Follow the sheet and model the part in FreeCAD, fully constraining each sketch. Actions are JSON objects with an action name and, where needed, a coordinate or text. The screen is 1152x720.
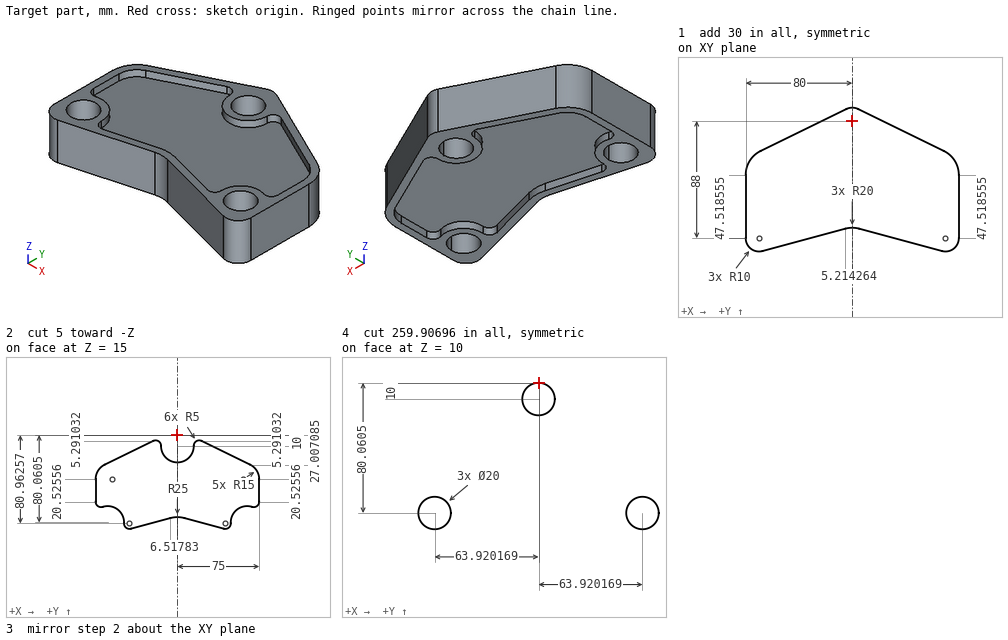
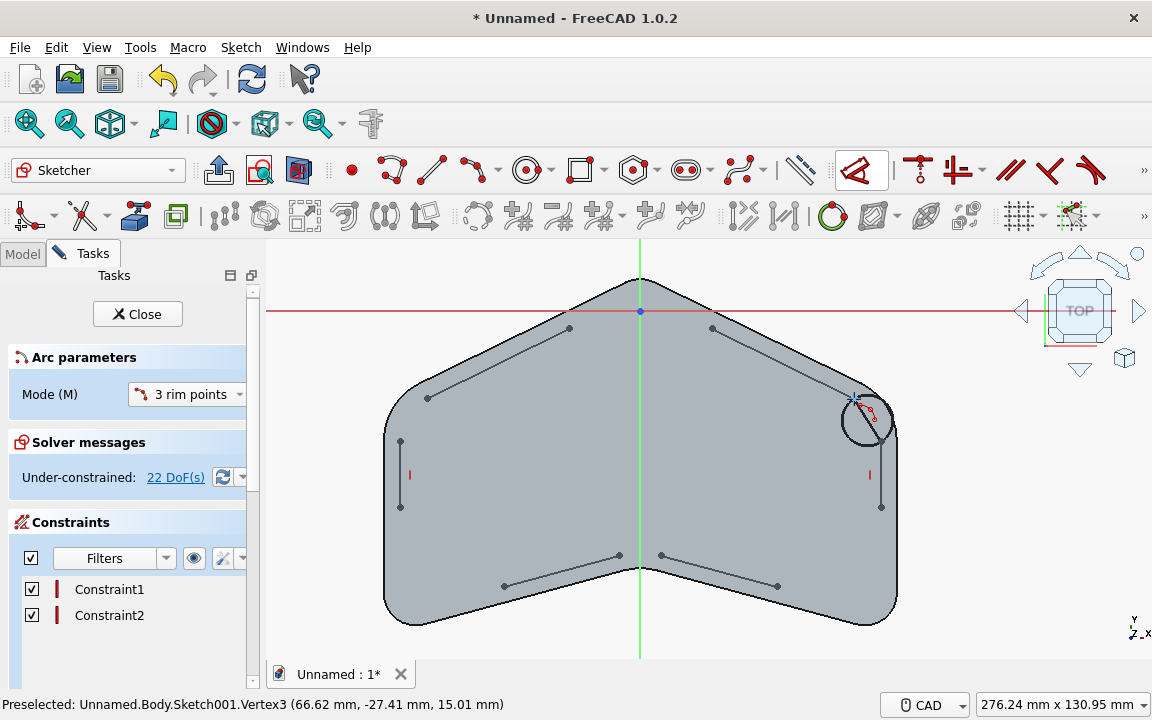
{"action": "scroll", "coordinate": [874, 415], "scroll_direction": "up", "scroll_amount": 4}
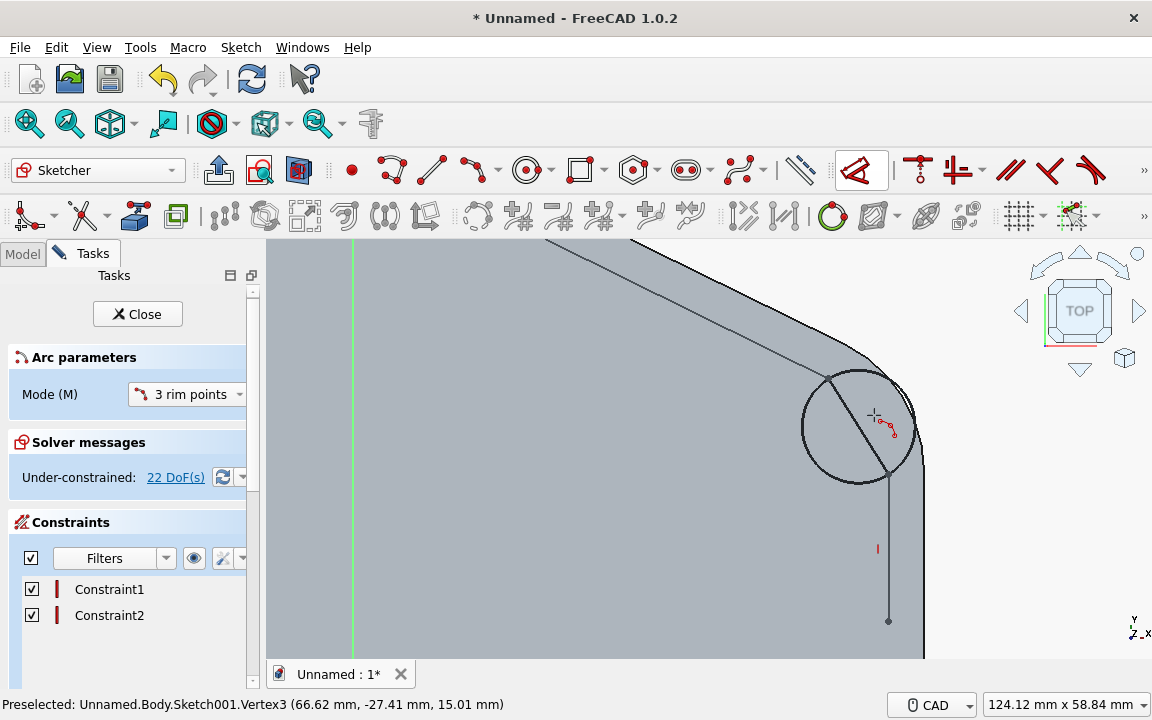
{"action": "left_click", "coordinate": [872, 416]}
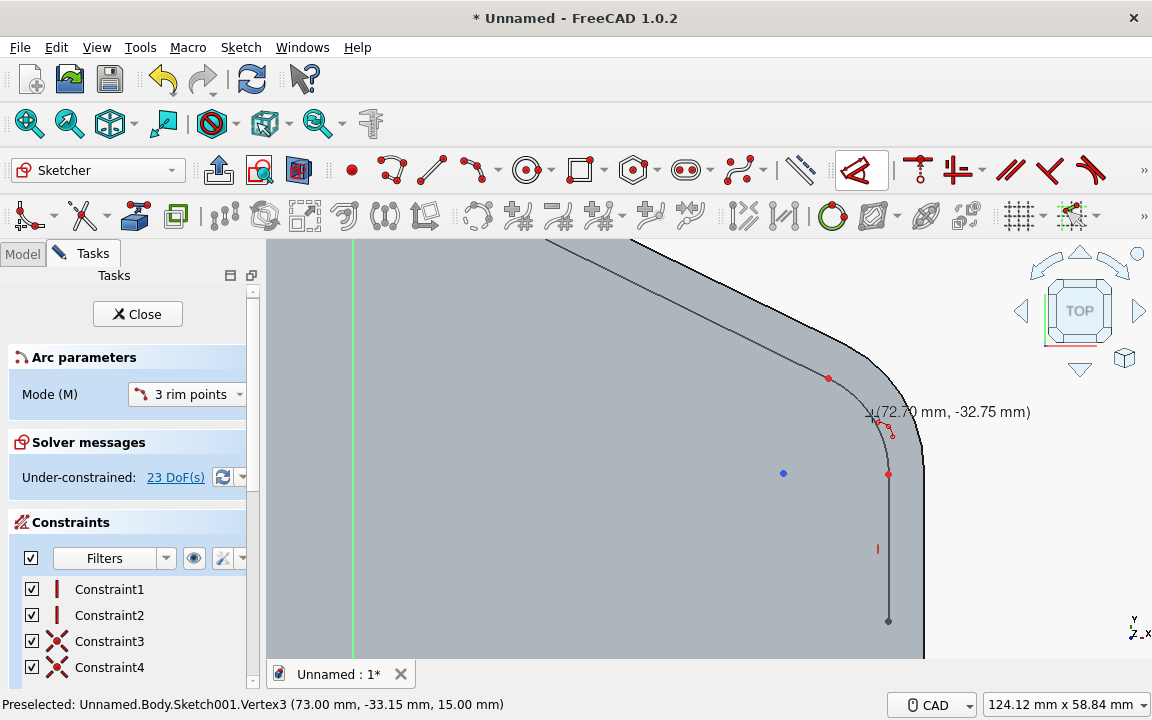
{"action": "scroll", "coordinate": [875, 416], "scroll_direction": "down", "scroll_amount": 4}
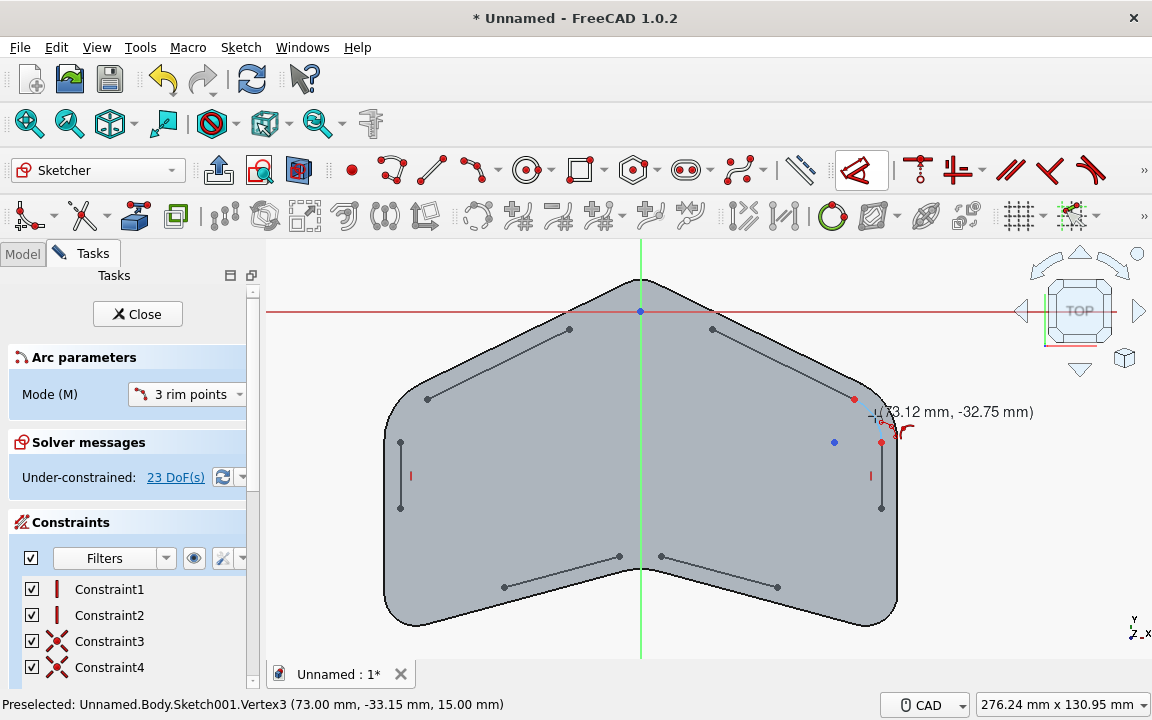
{"action": "left_click", "coordinate": [713, 330]}
{"action": "left_click", "coordinate": [689, 343]}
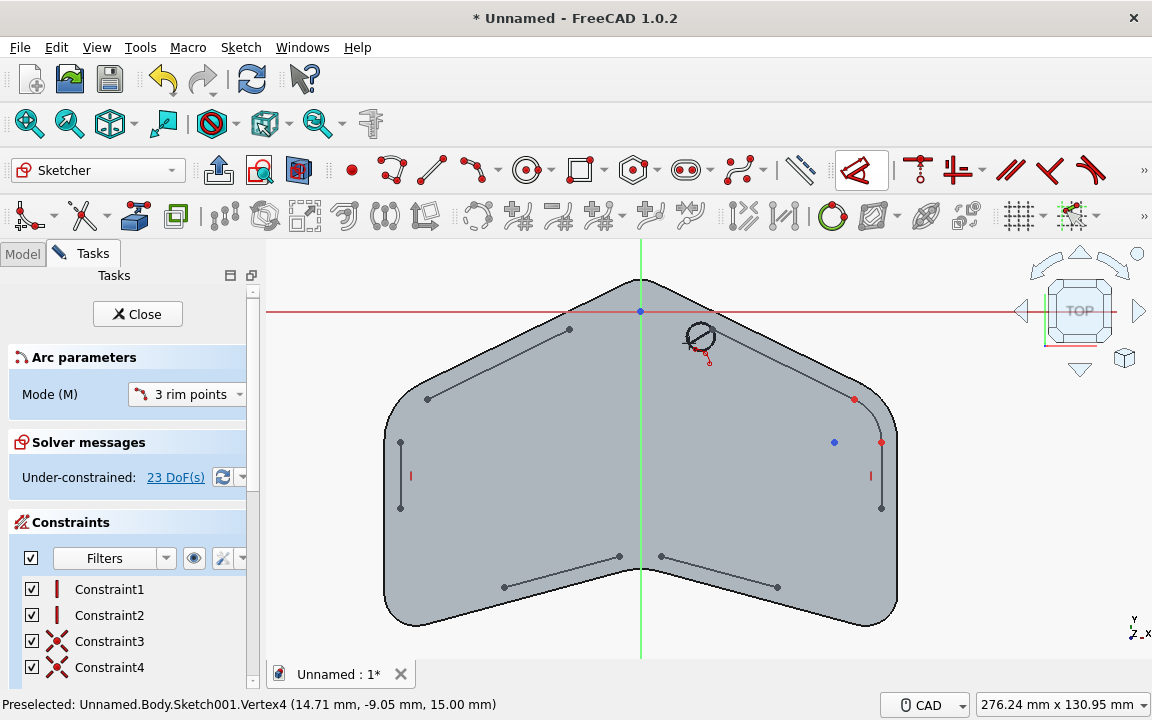
{"action": "scroll", "coordinate": [696, 329], "scroll_direction": "up", "scroll_amount": 4}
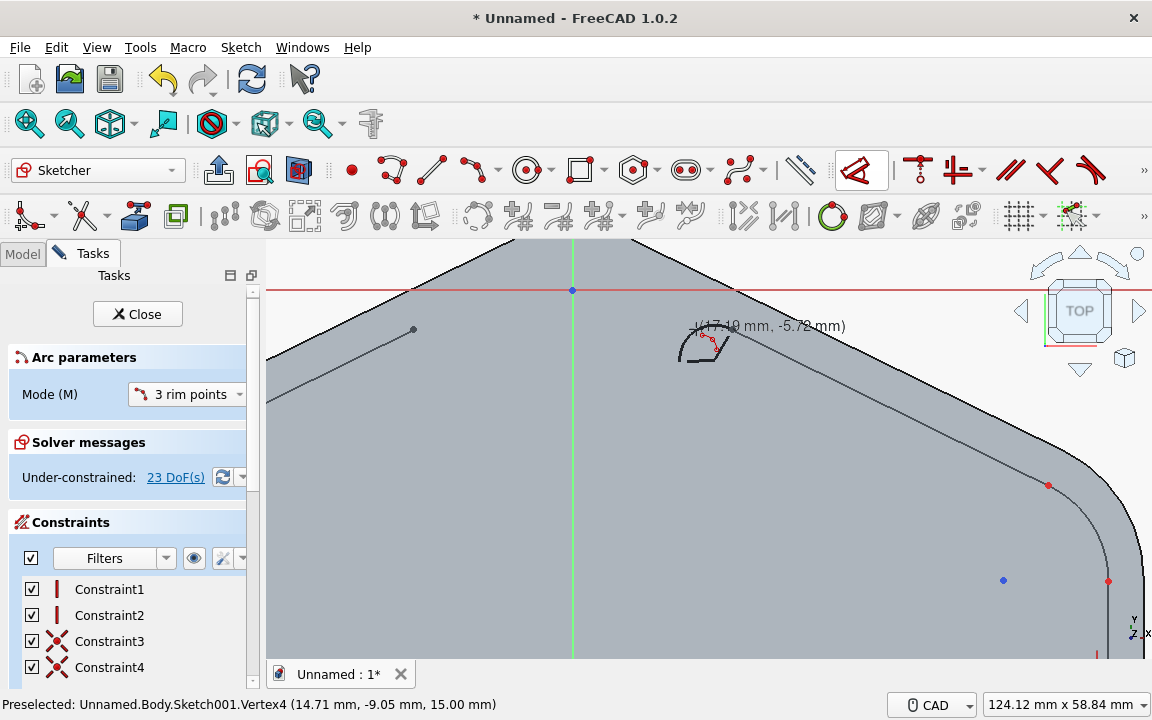
{"action": "left_click", "coordinate": [696, 330]}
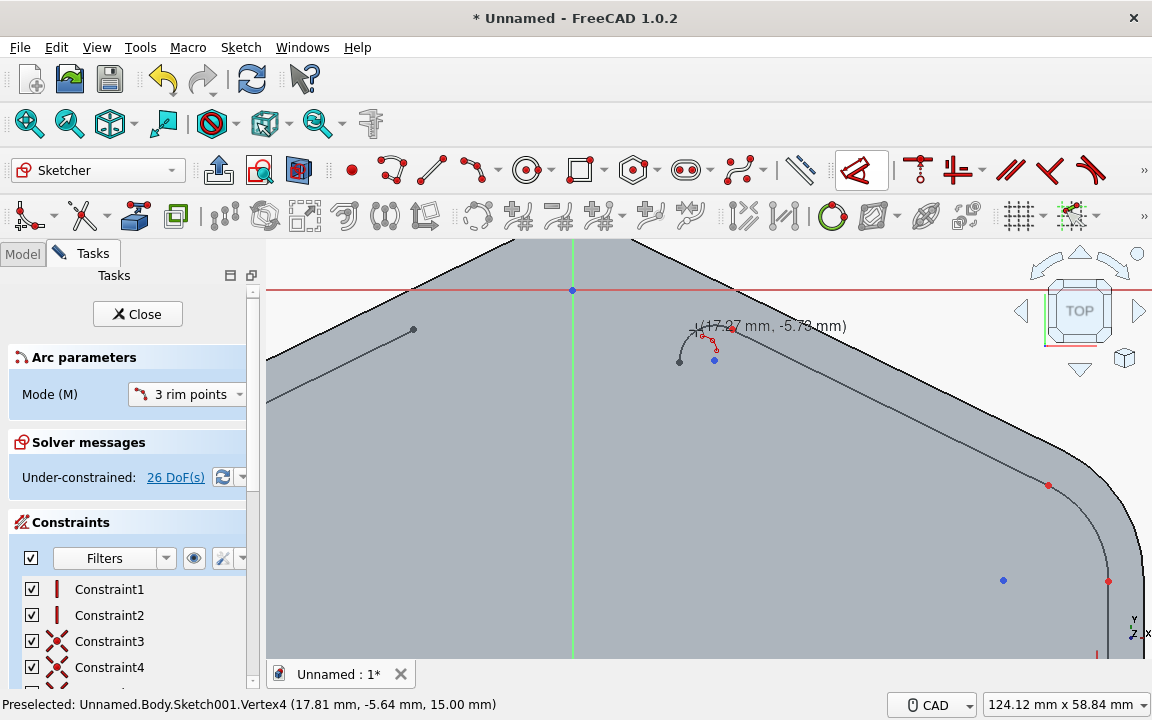
{"action": "left_click", "coordinate": [680, 362]}
{"action": "left_click", "coordinate": [466, 360]}
{"action": "left_click", "coordinate": [539, 463]}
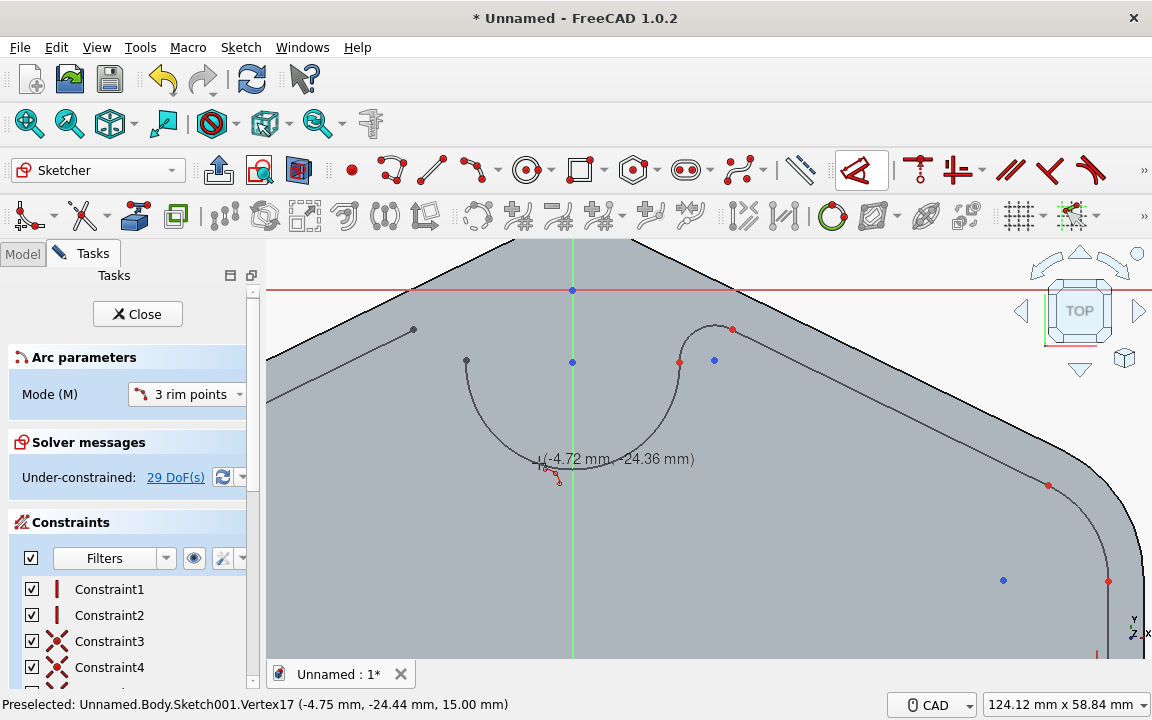
{"action": "left_click", "coordinate": [466, 361]}
{"action": "left_click", "coordinate": [414, 330]}
{"action": "left_click", "coordinate": [449, 330]}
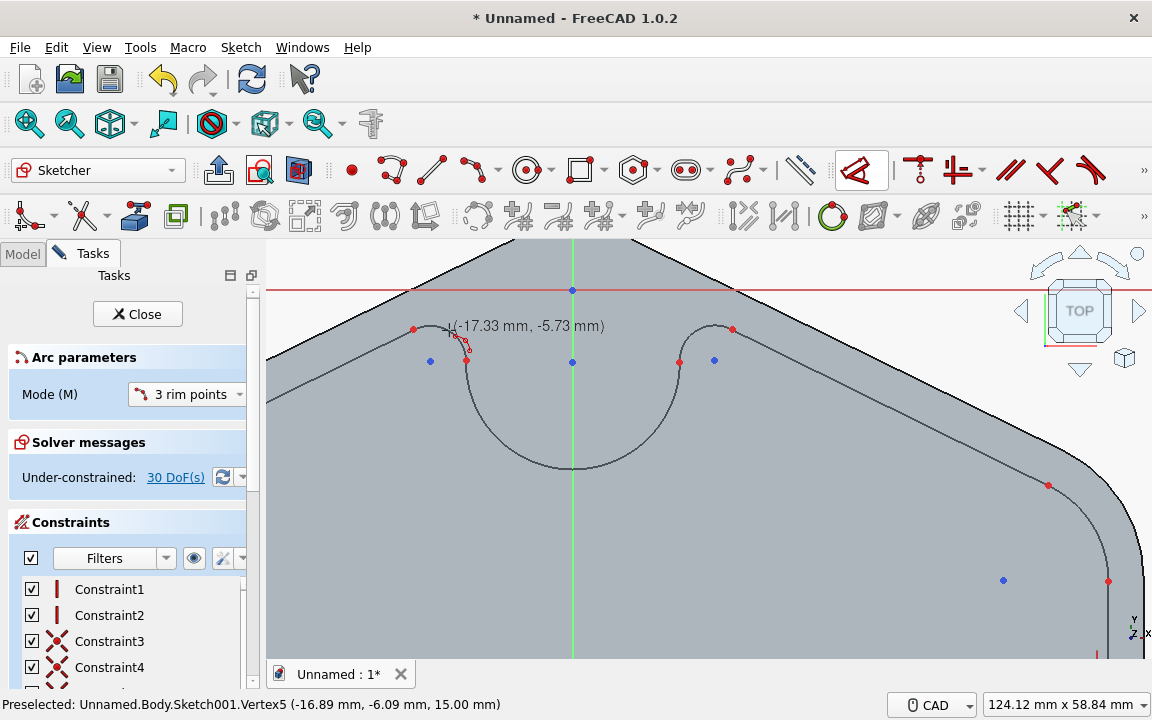
{"action": "scroll", "coordinate": [696, 329], "scroll_direction": "down", "scroll_amount": 4}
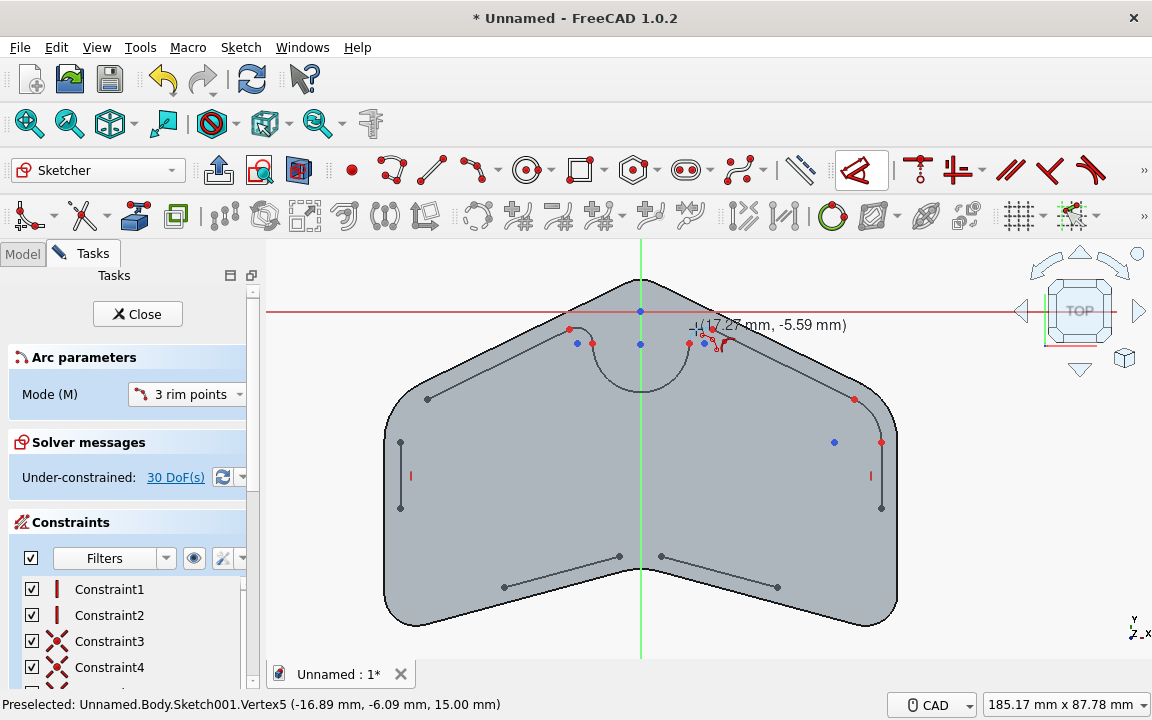
{"action": "left_click", "coordinate": [428, 400]}
{"action": "left_click", "coordinate": [401, 443]}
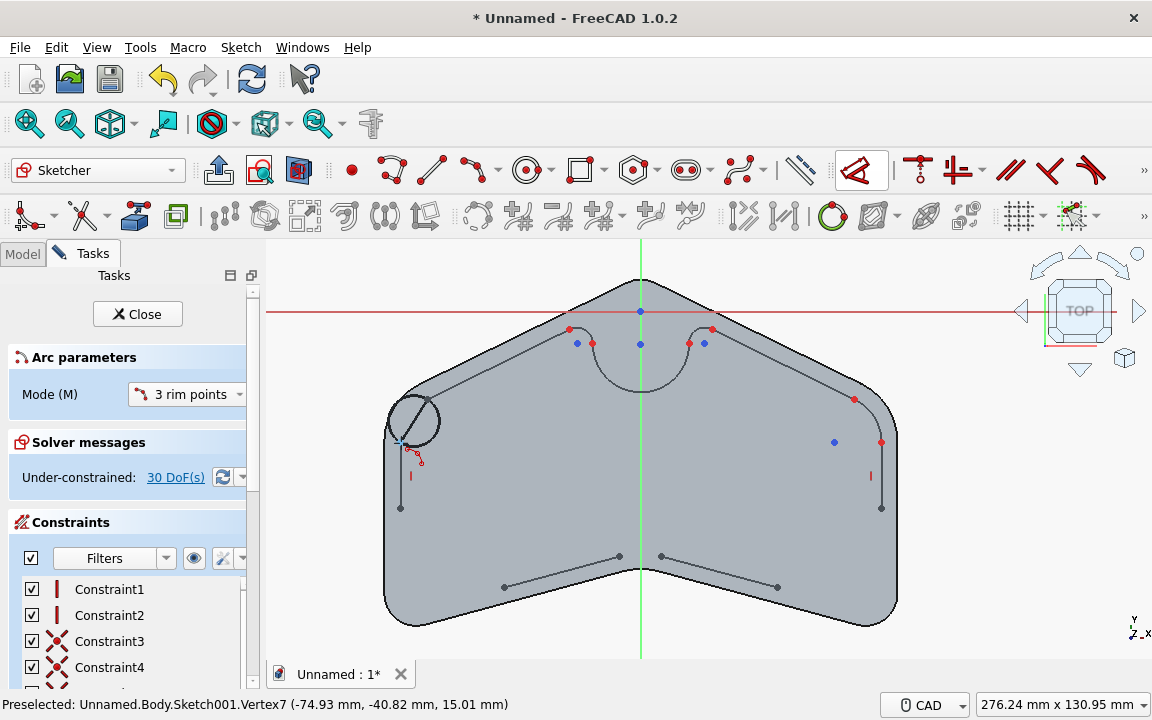
{"action": "scroll", "coordinate": [408, 416], "scroll_direction": "up", "scroll_amount": 4}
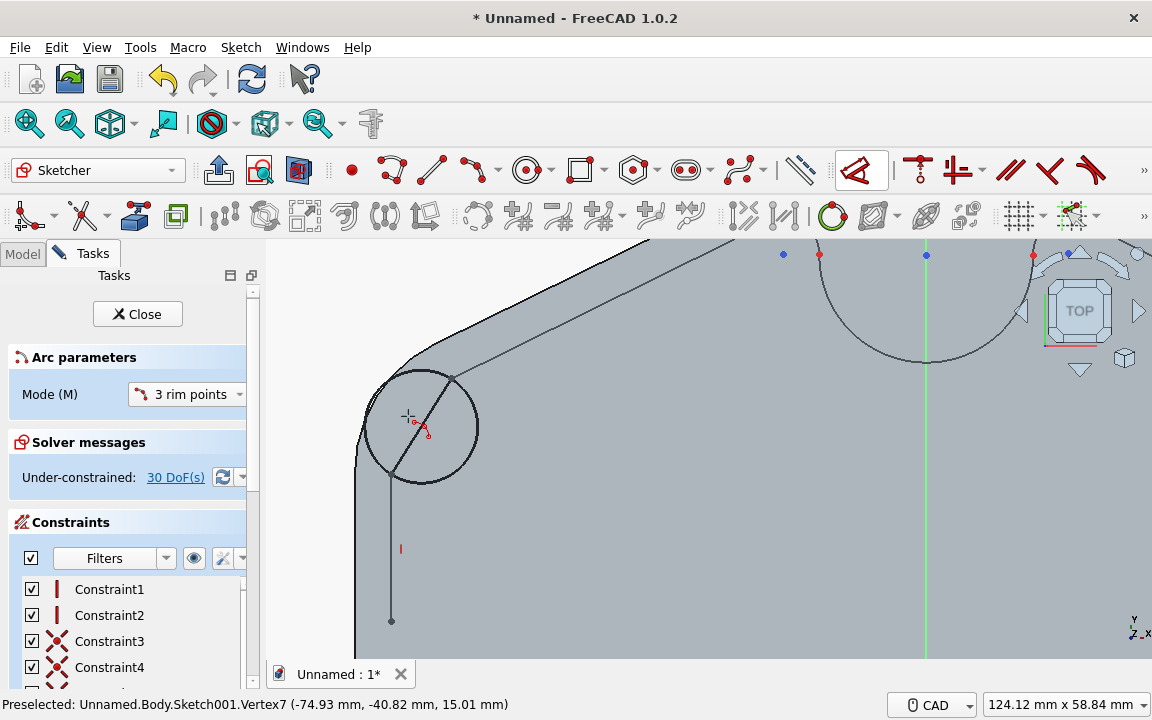
{"action": "left_click", "coordinate": [407, 416]}